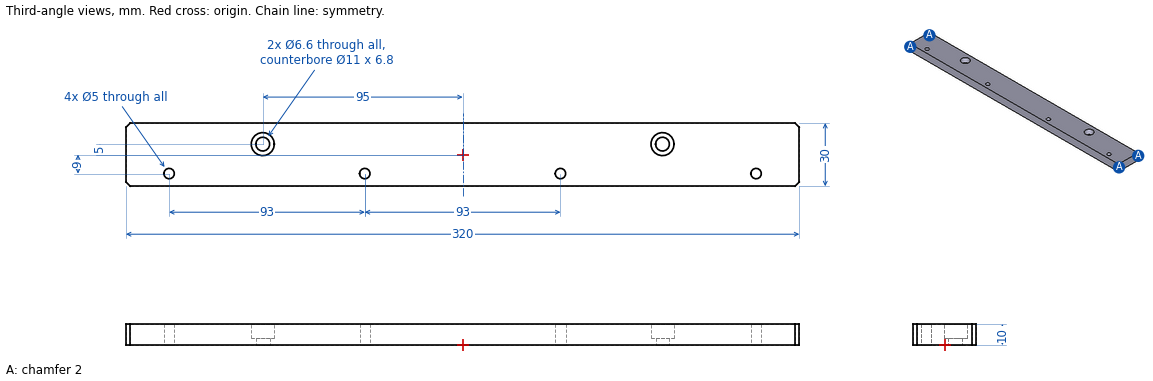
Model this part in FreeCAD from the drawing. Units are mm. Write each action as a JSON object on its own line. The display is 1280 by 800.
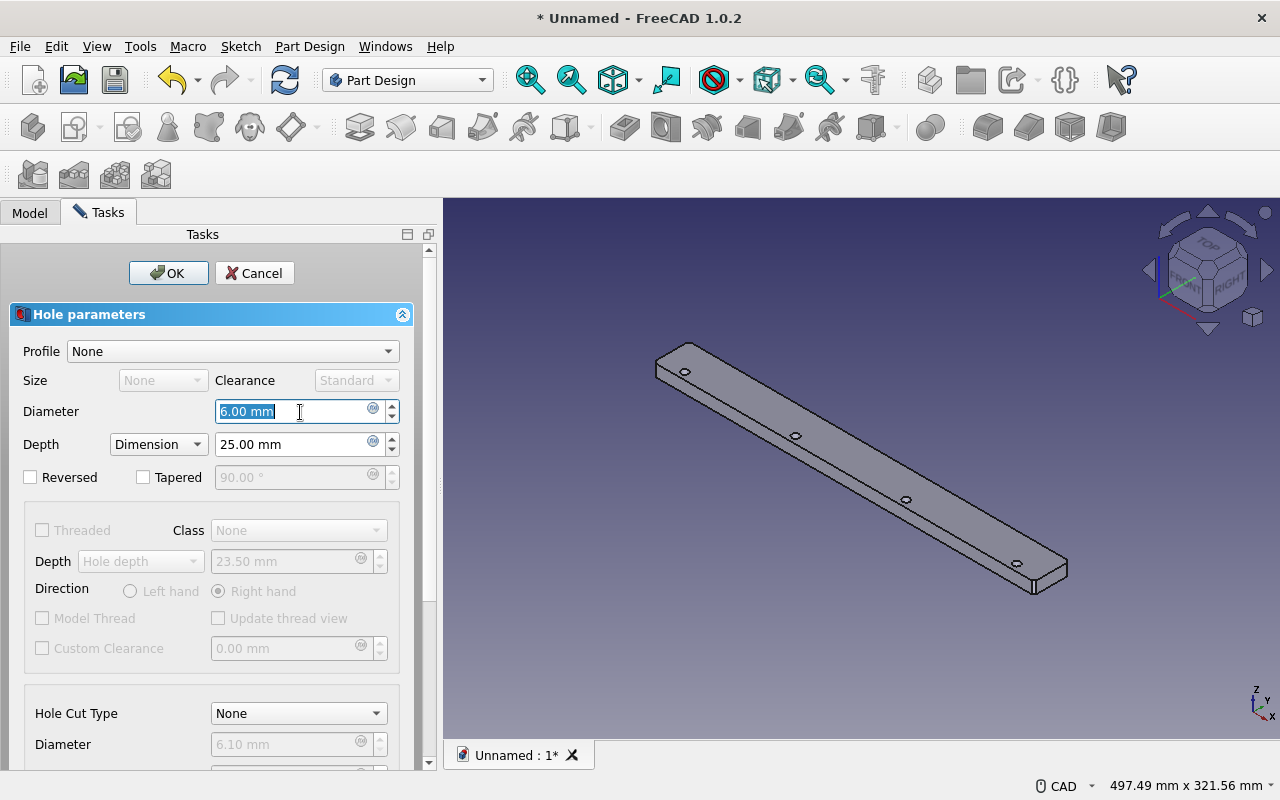
{"action": "type", "text": "5"}
{"action": "key", "text": "Tab"}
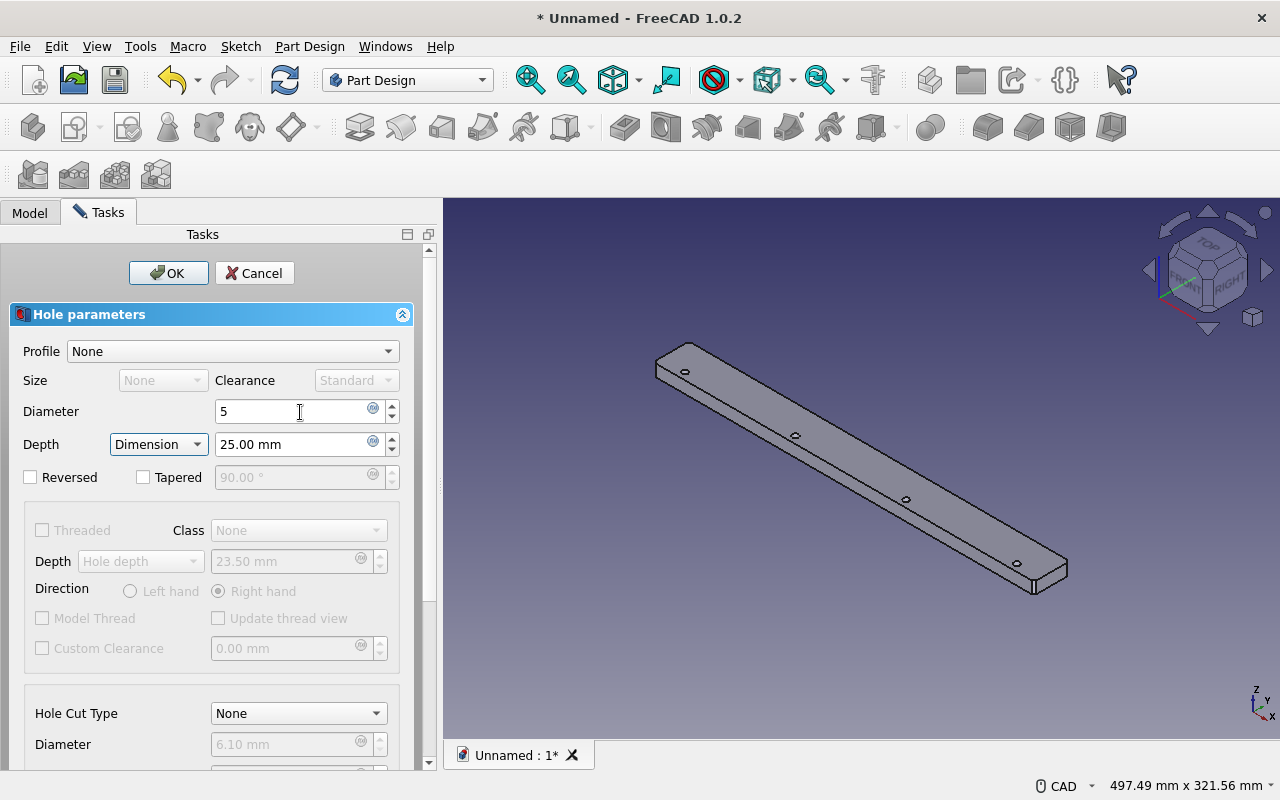
{"action": "left_click", "coordinate": [160, 444]}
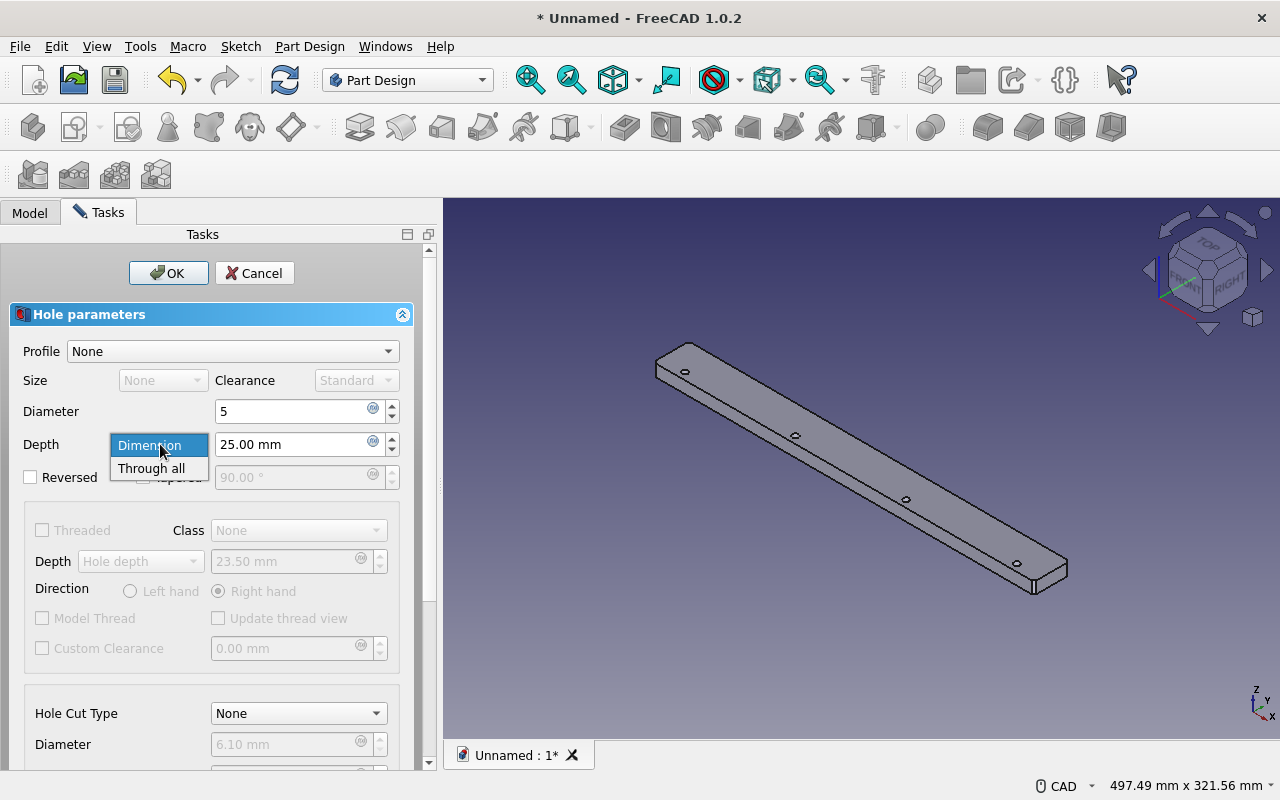
{"action": "left_click", "coordinate": [158, 468]}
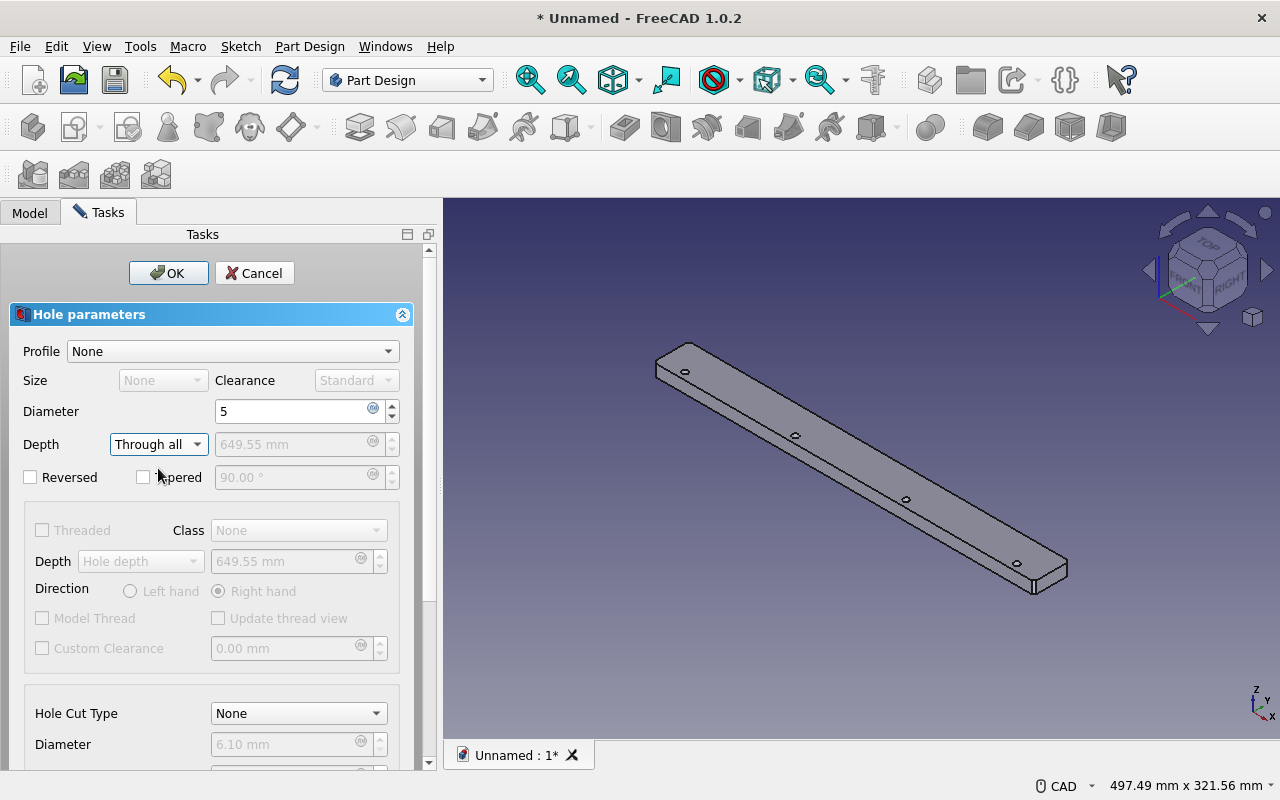
{"action": "left_click", "coordinate": [169, 273]}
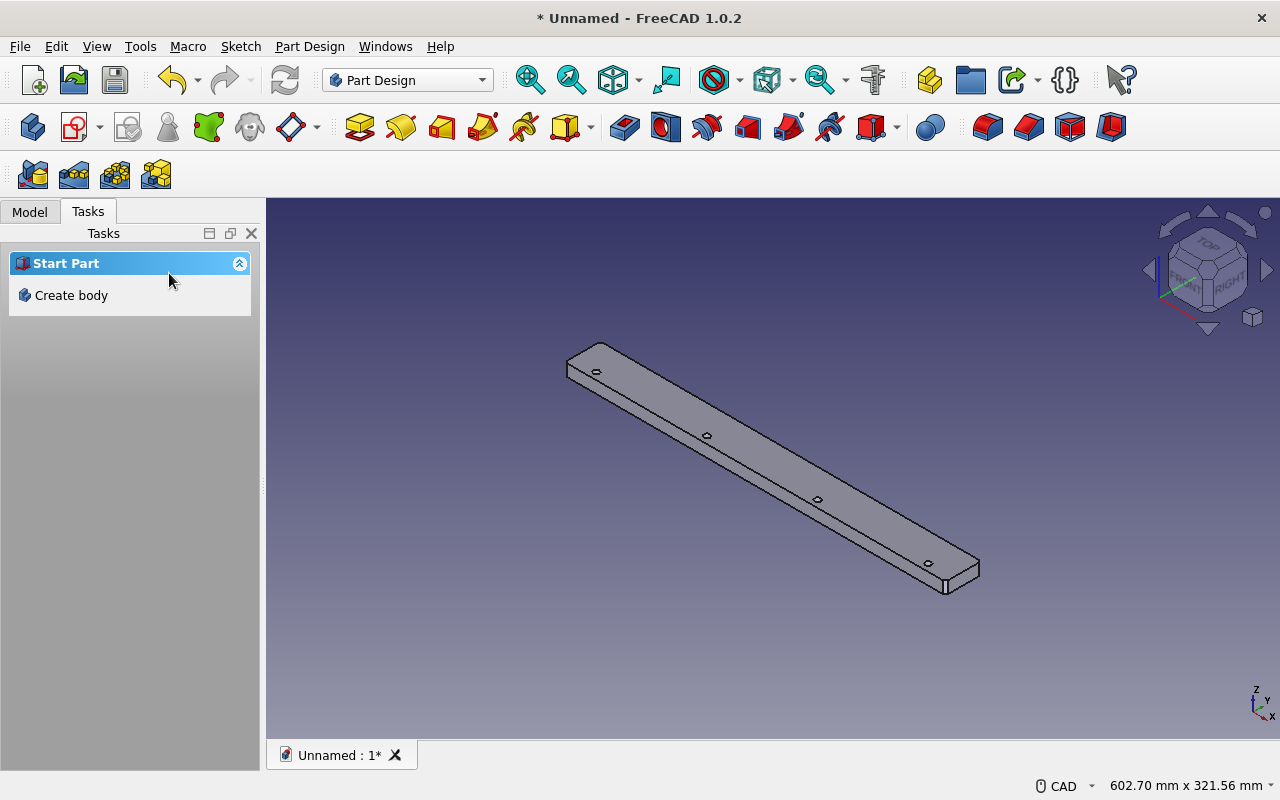
{"action": "left_click", "coordinate": [882, 523]}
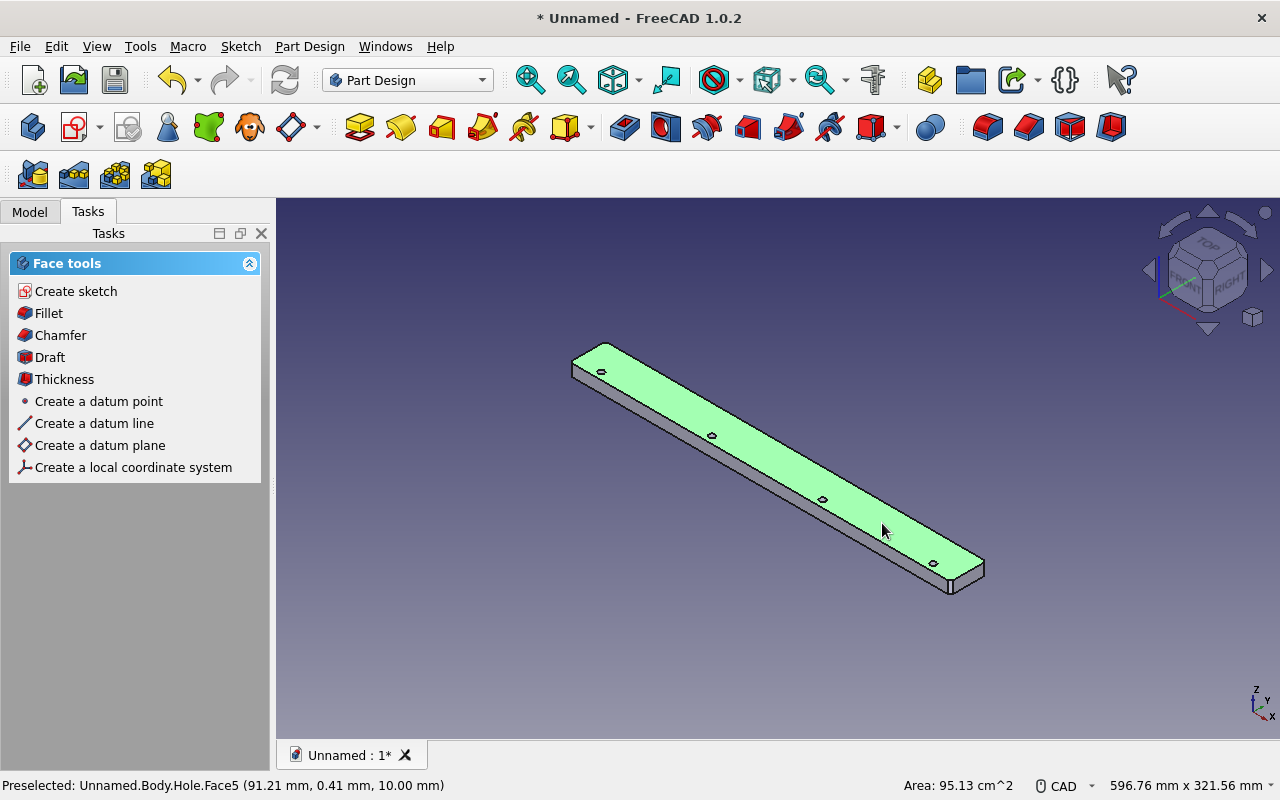
{"action": "left_click", "coordinate": [74, 128]}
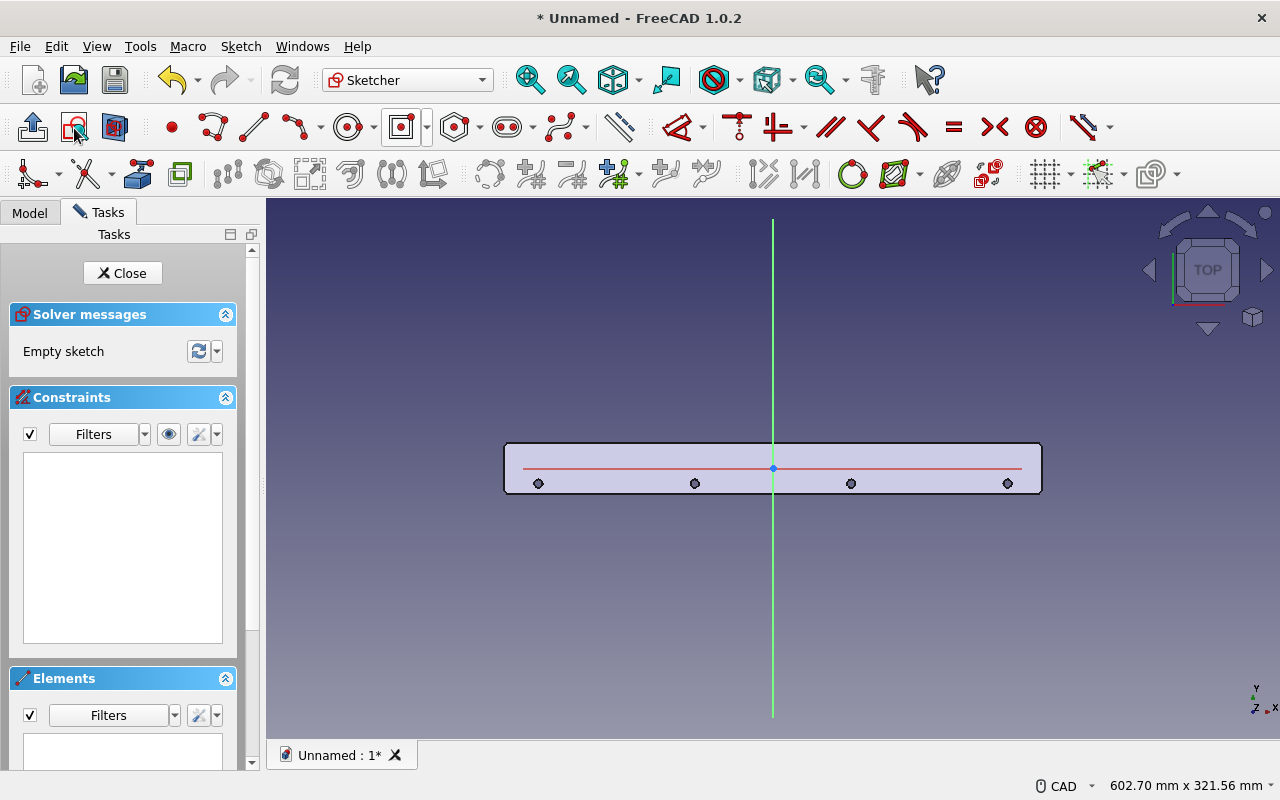
{"action": "scroll", "coordinate": [856, 453], "scroll_direction": "up", "scroll_amount": 3}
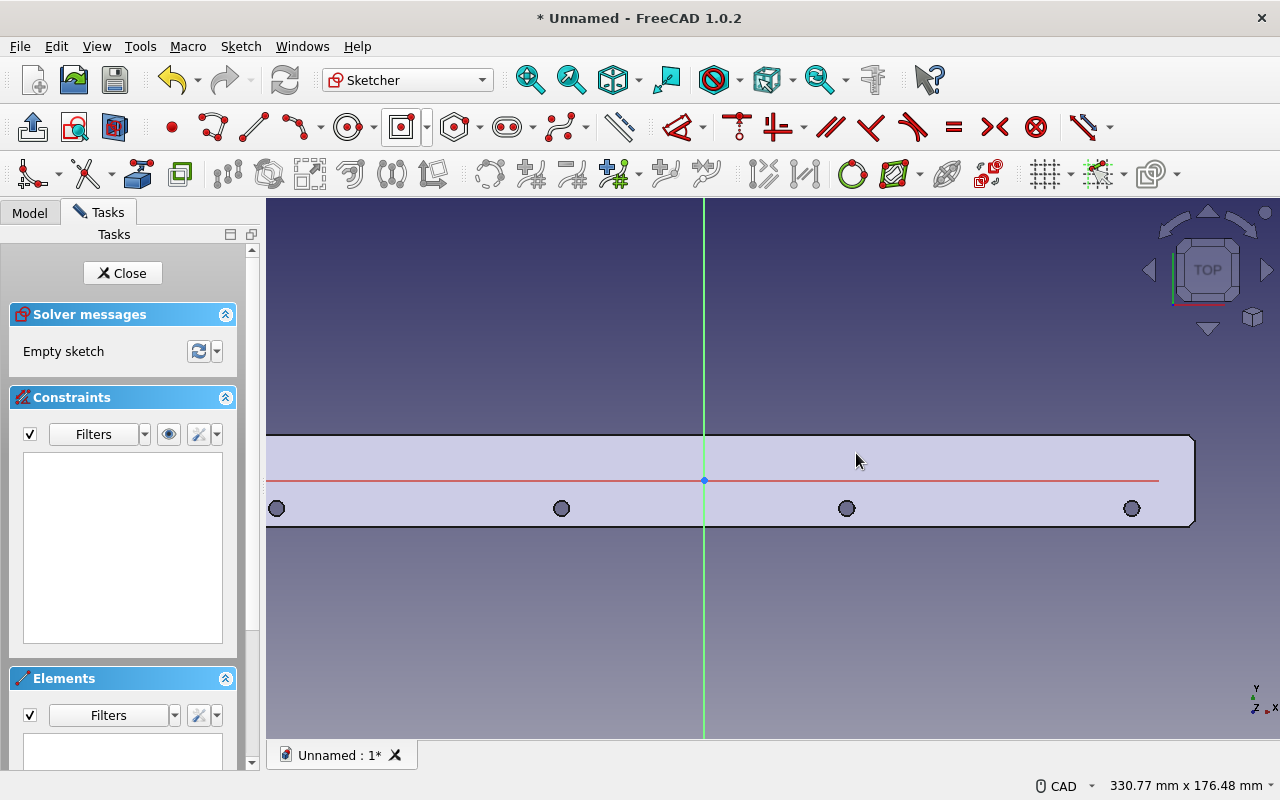
{"action": "left_click", "coordinate": [348, 128]}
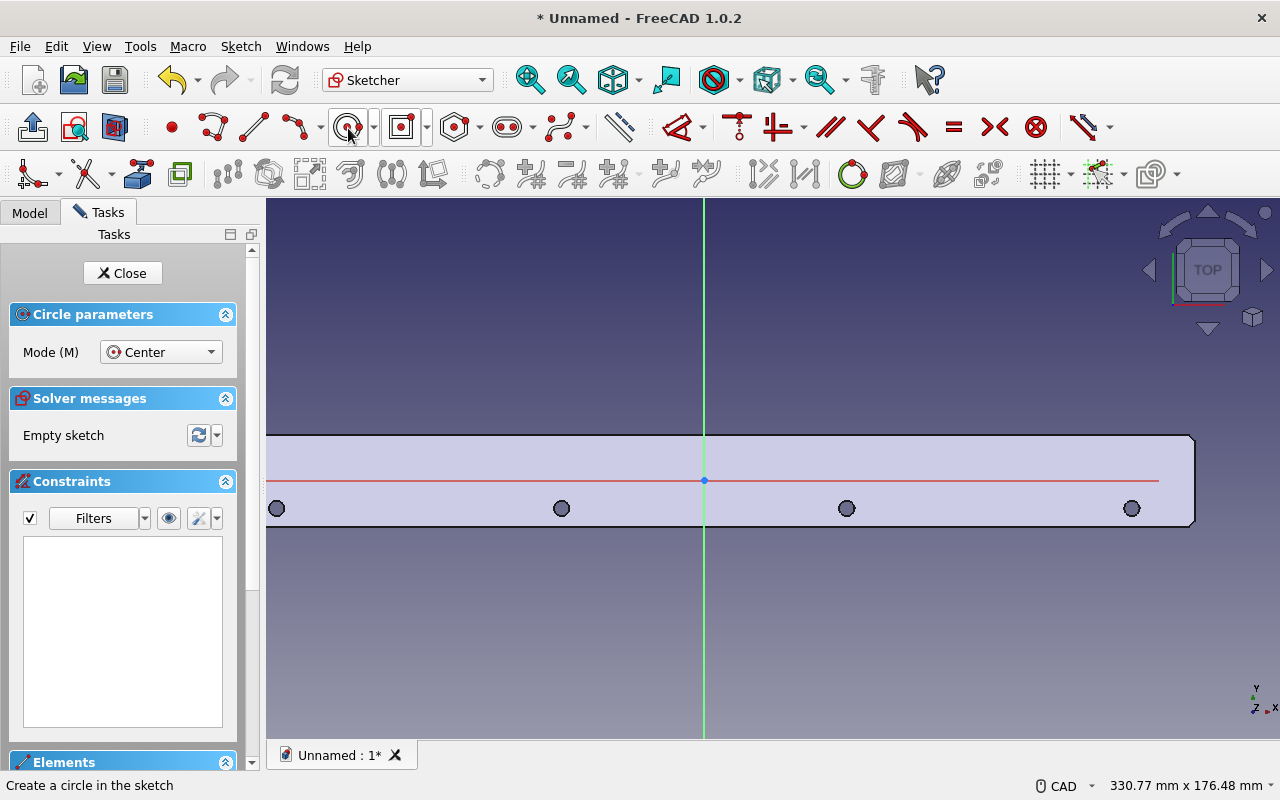
{"action": "scroll", "coordinate": [413, 466], "scroll_direction": "up", "scroll_amount": 5}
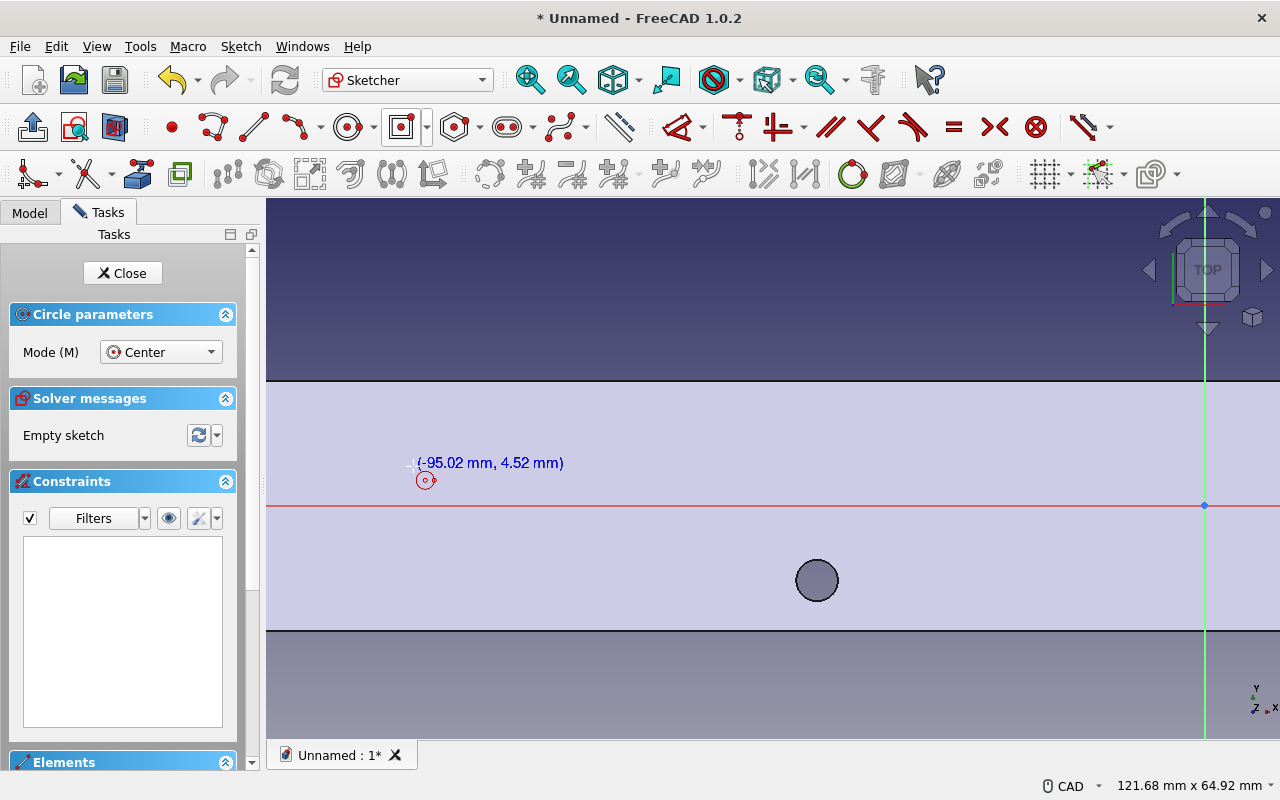
{"action": "left_click", "coordinate": [413, 464]}
{"action": "left_click", "coordinate": [432, 444]}